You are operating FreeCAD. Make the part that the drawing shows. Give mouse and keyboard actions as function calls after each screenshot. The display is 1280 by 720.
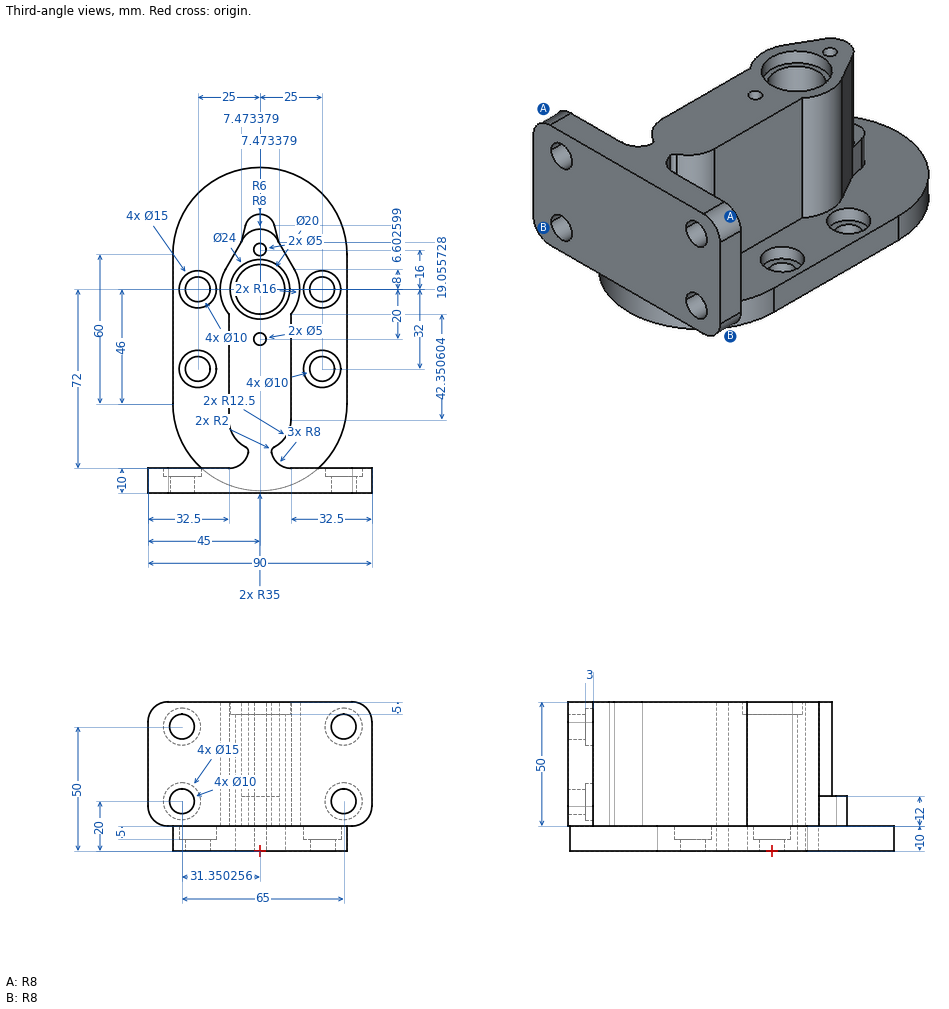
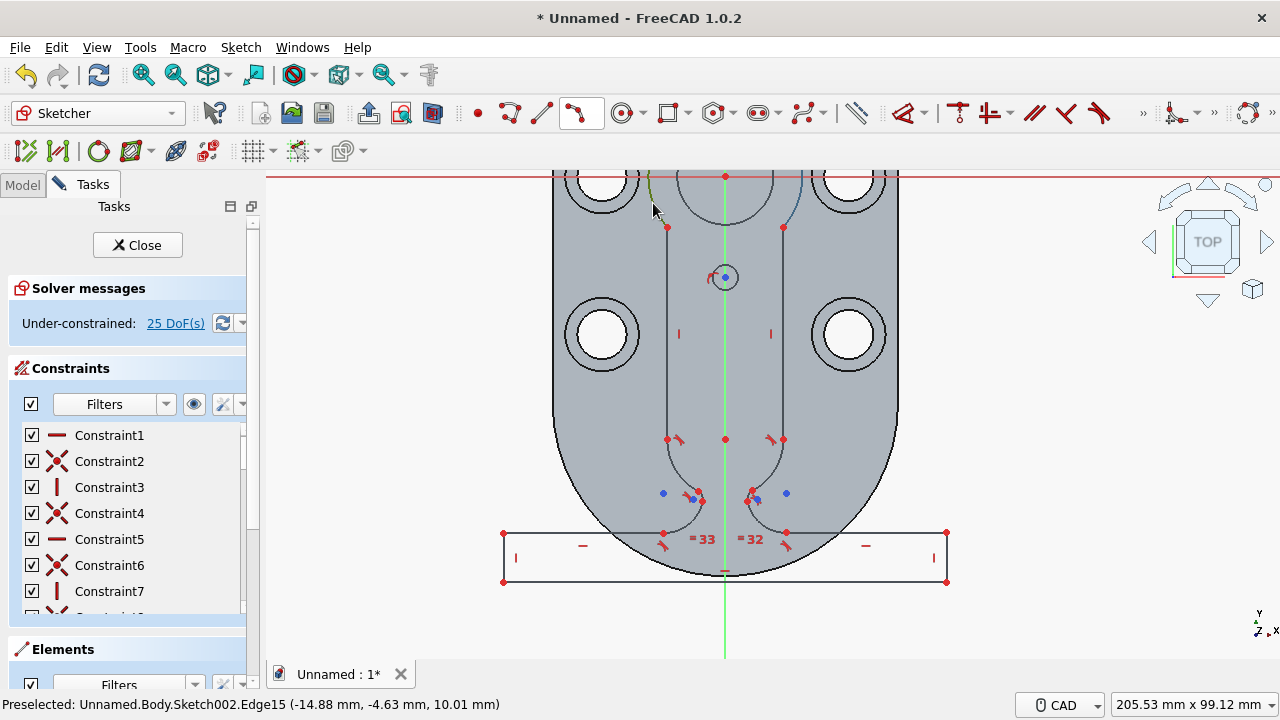
key(e)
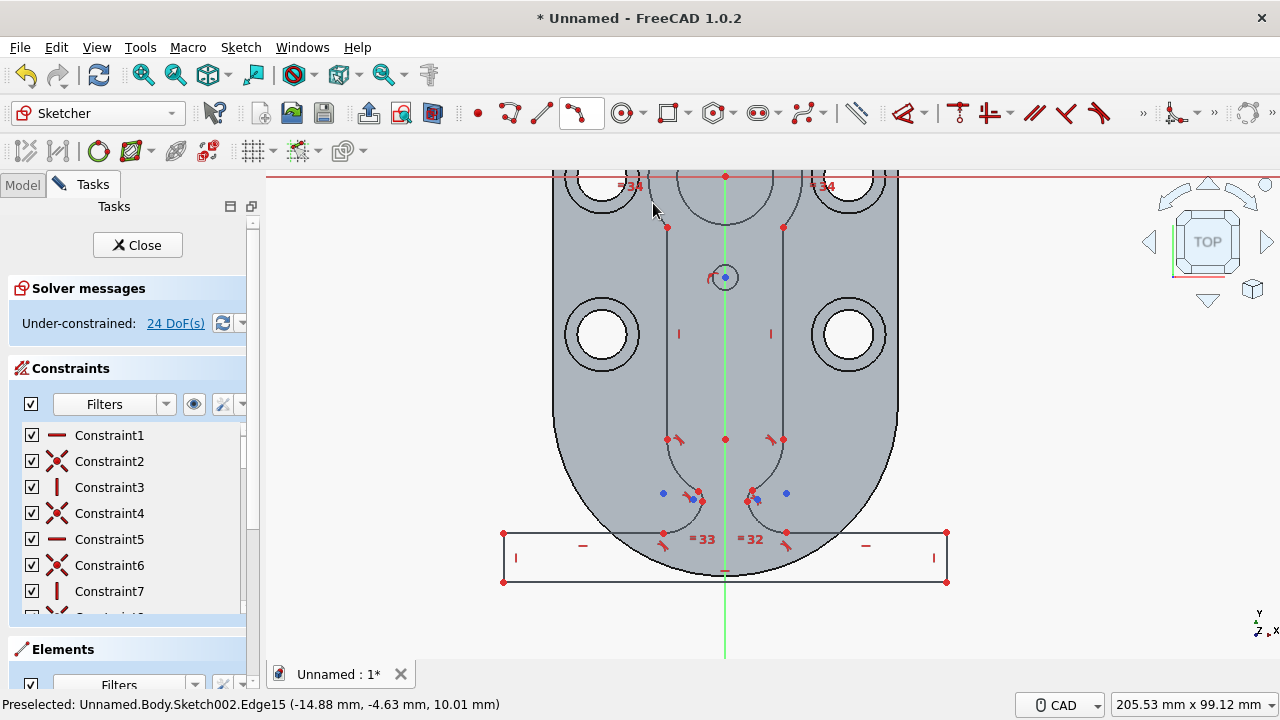
click(768, 479)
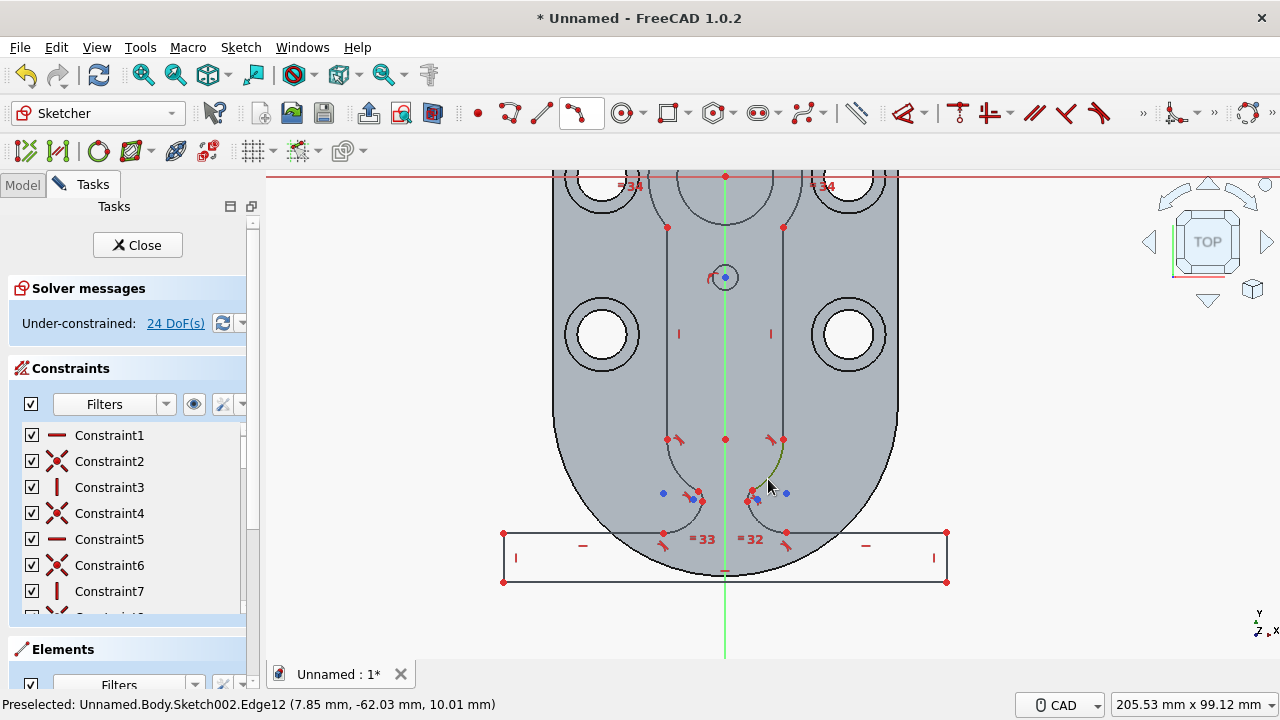
click(670, 458)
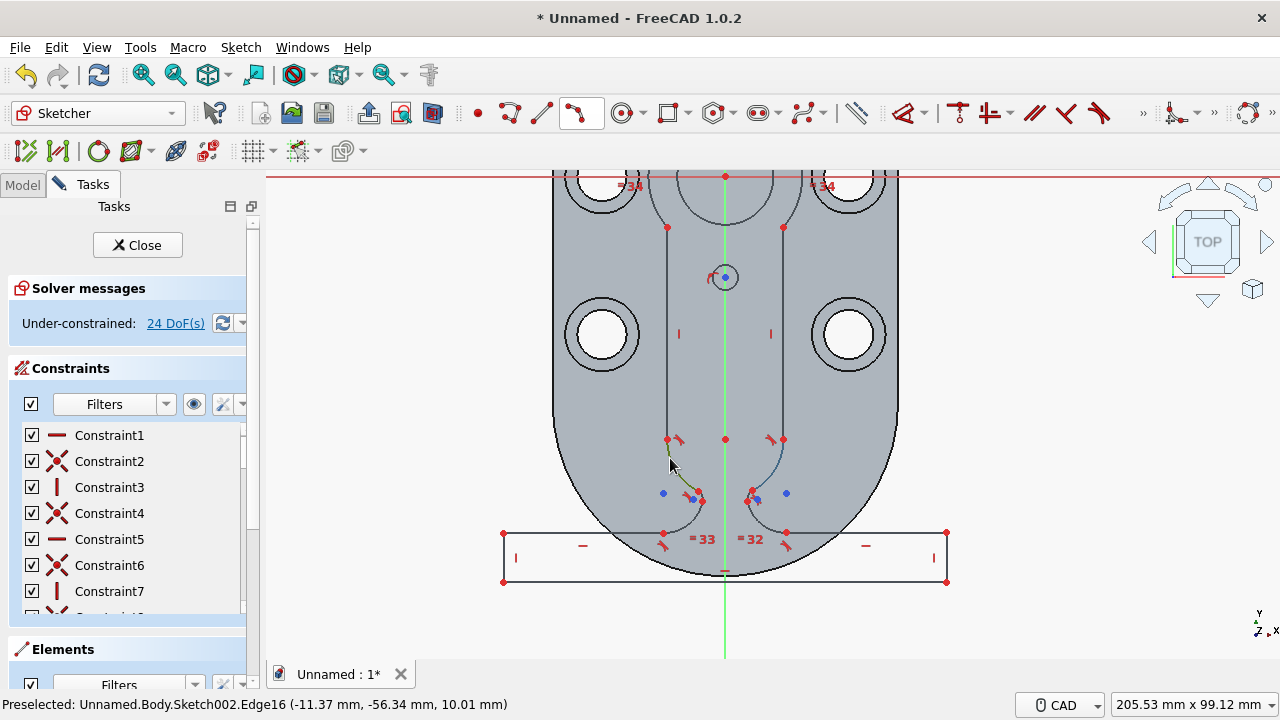
key(e)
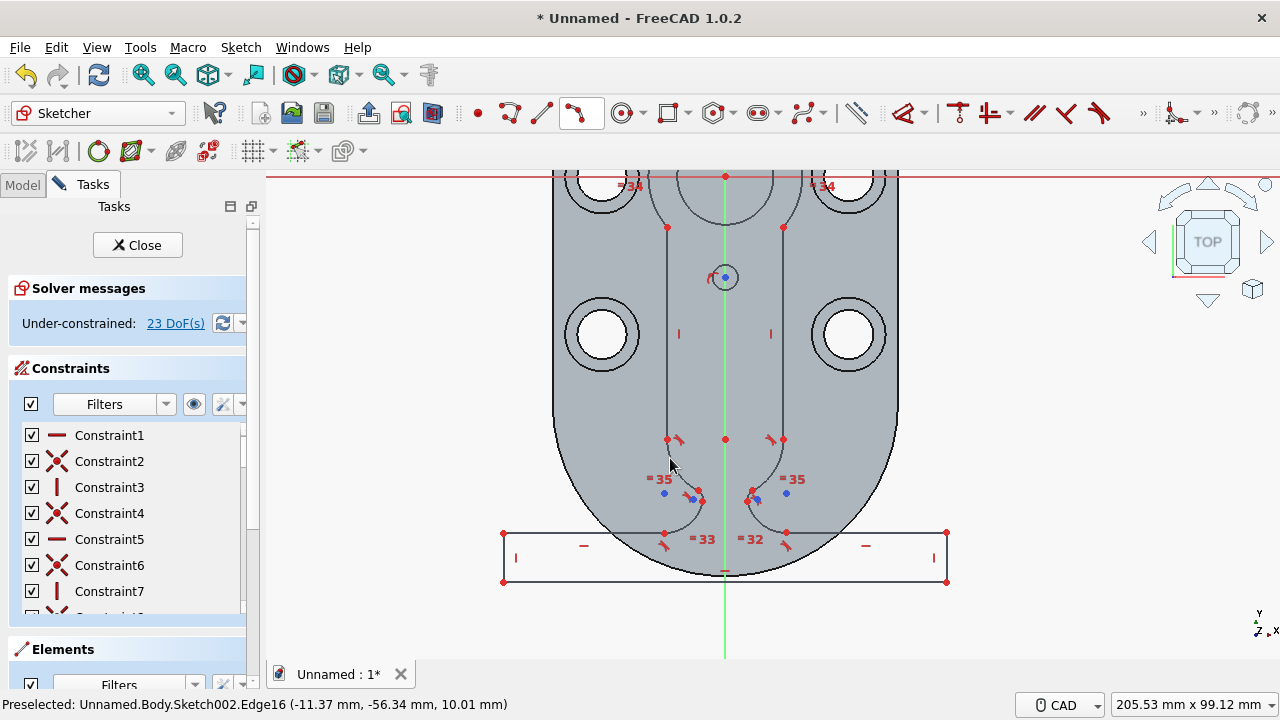
scroll(748, 495, up, 4)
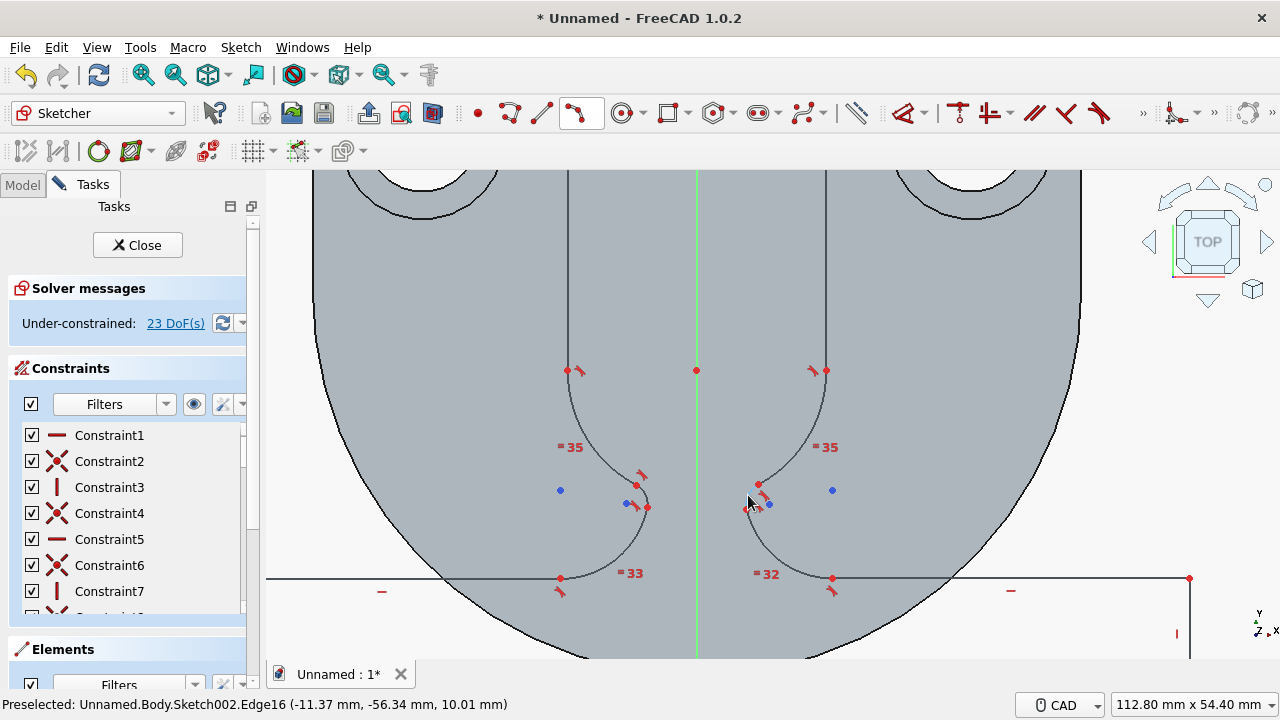
click(748, 495)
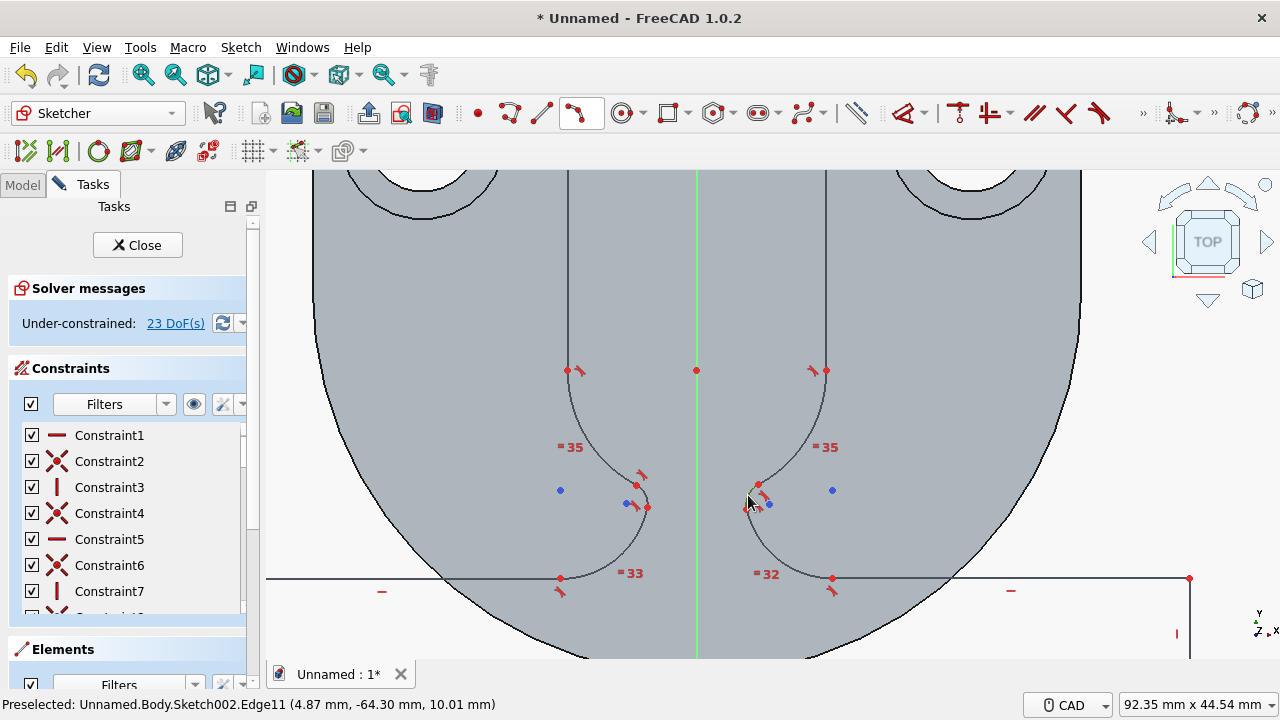
click(646, 495)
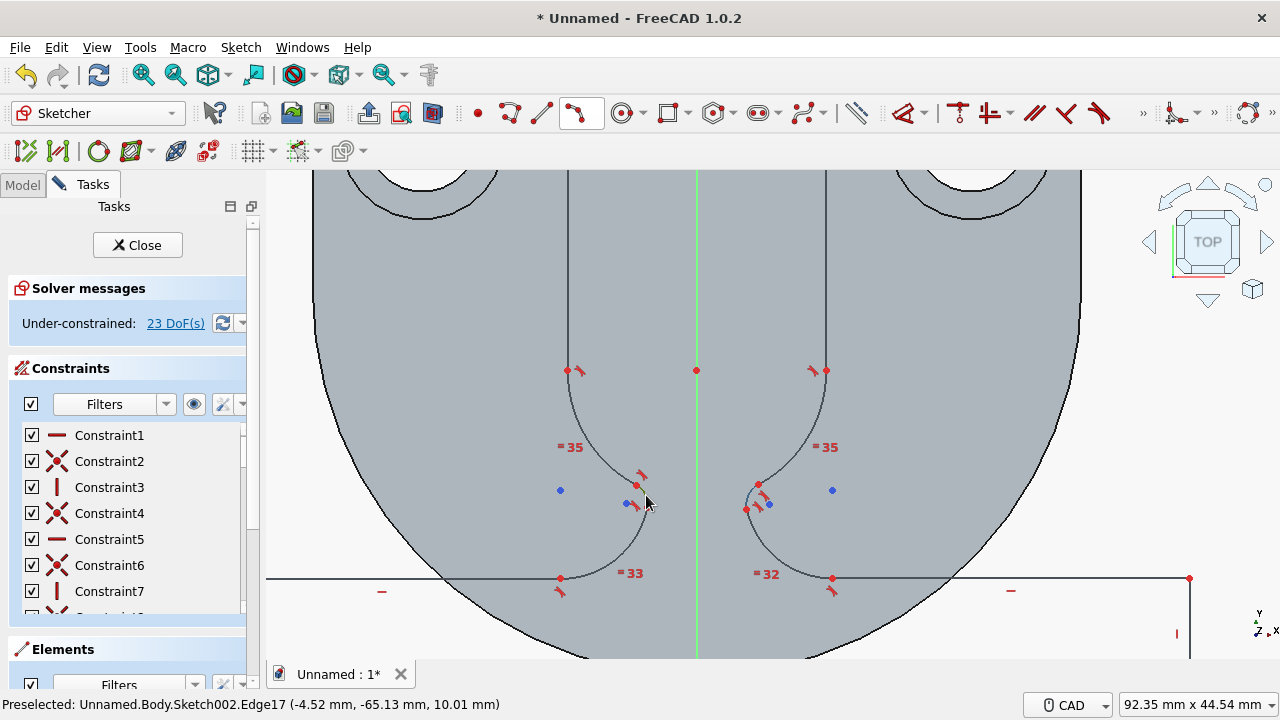
key(e)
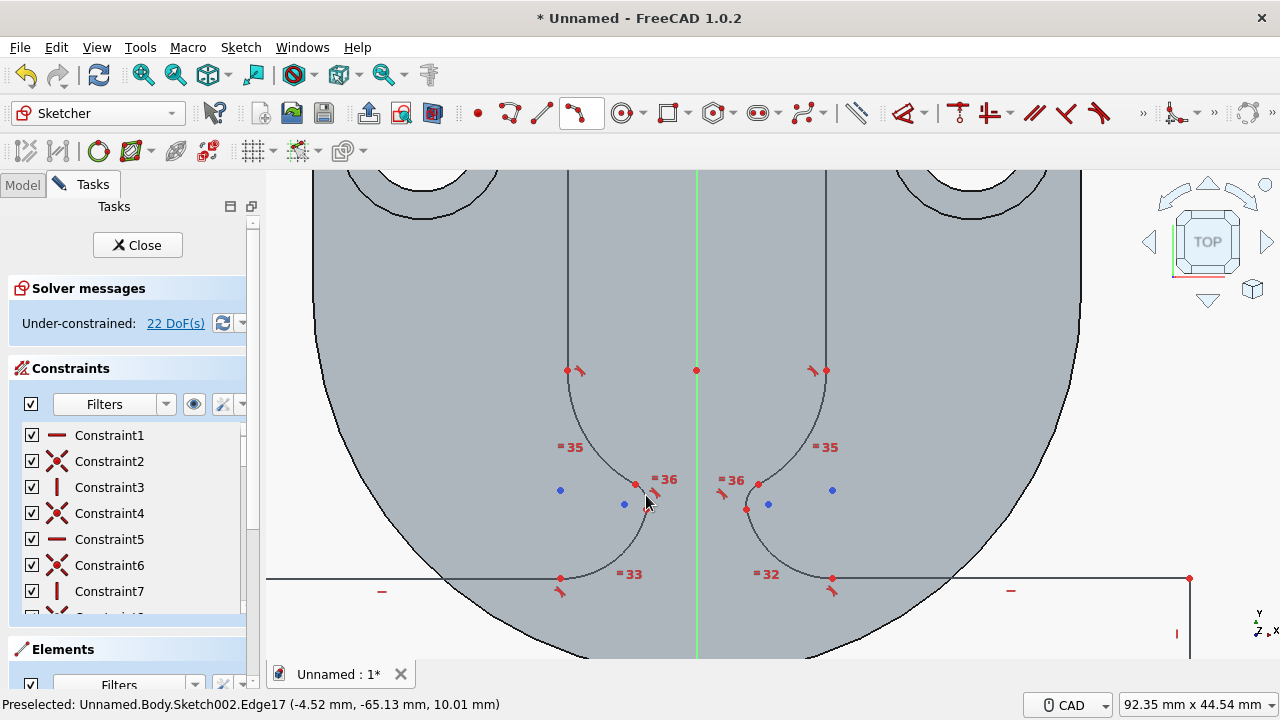
scroll(707, 516, down, 7)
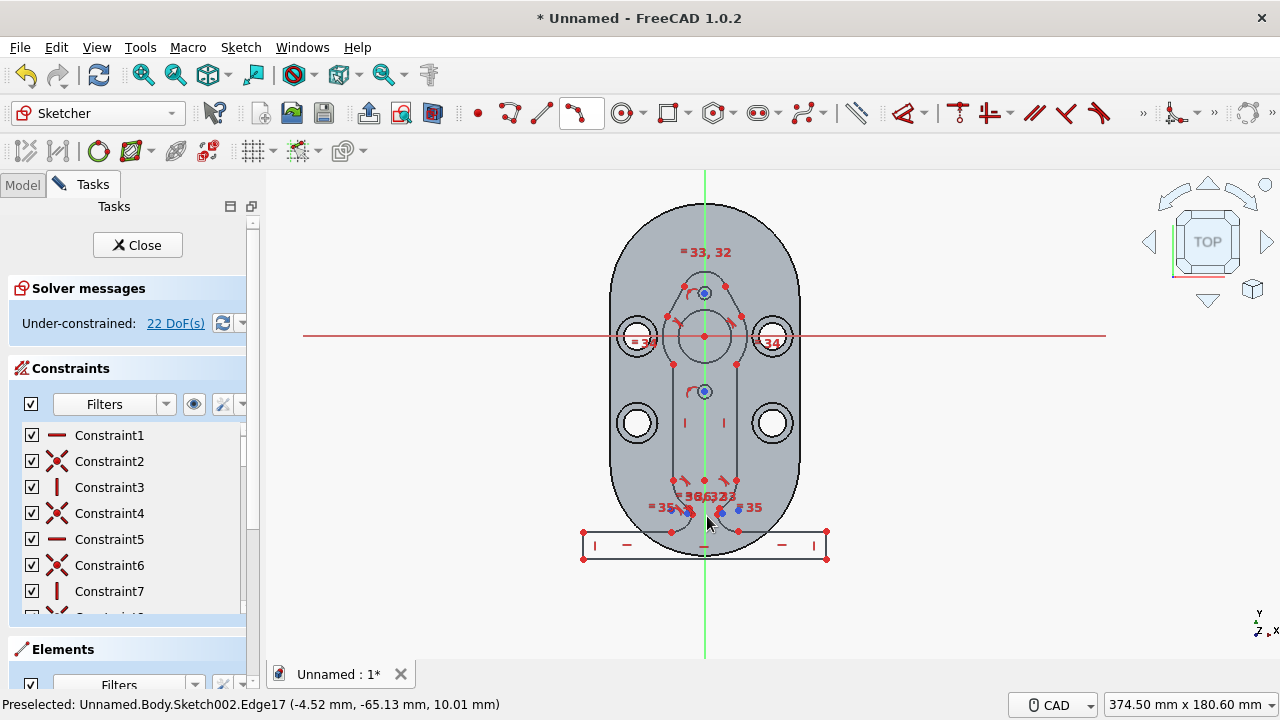
scroll(710, 387, up, 6)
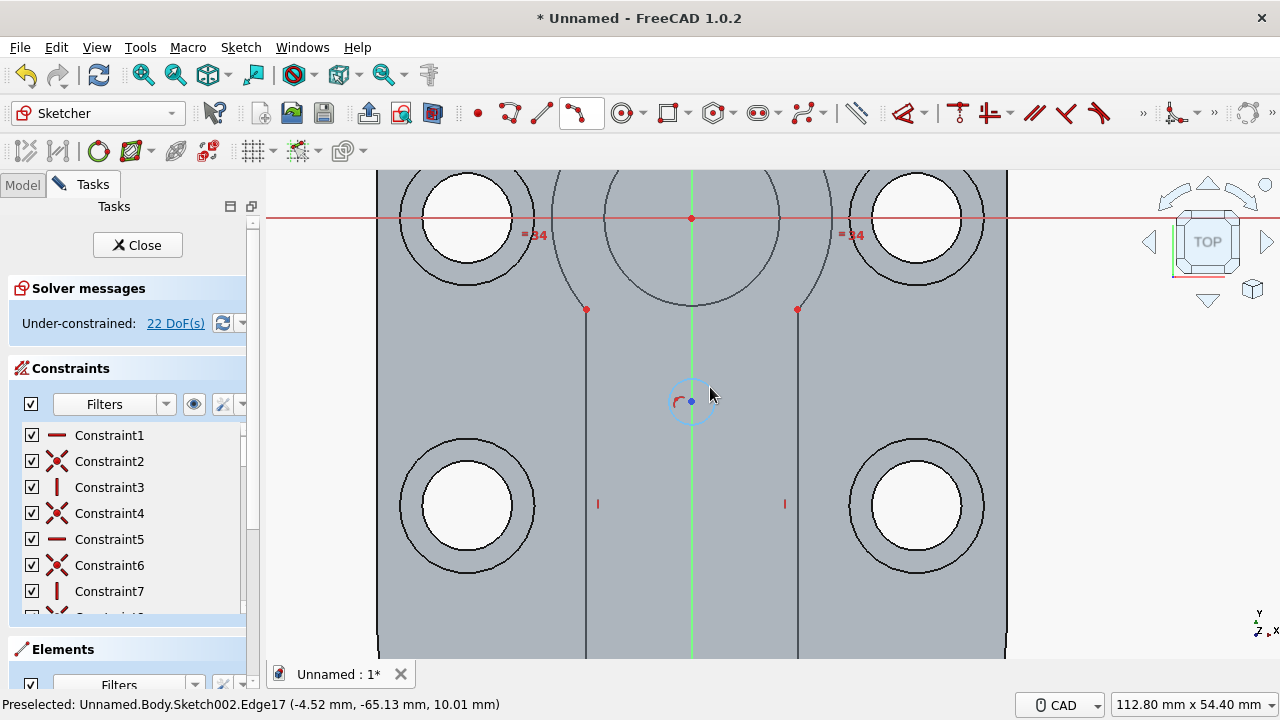
click(708, 386)